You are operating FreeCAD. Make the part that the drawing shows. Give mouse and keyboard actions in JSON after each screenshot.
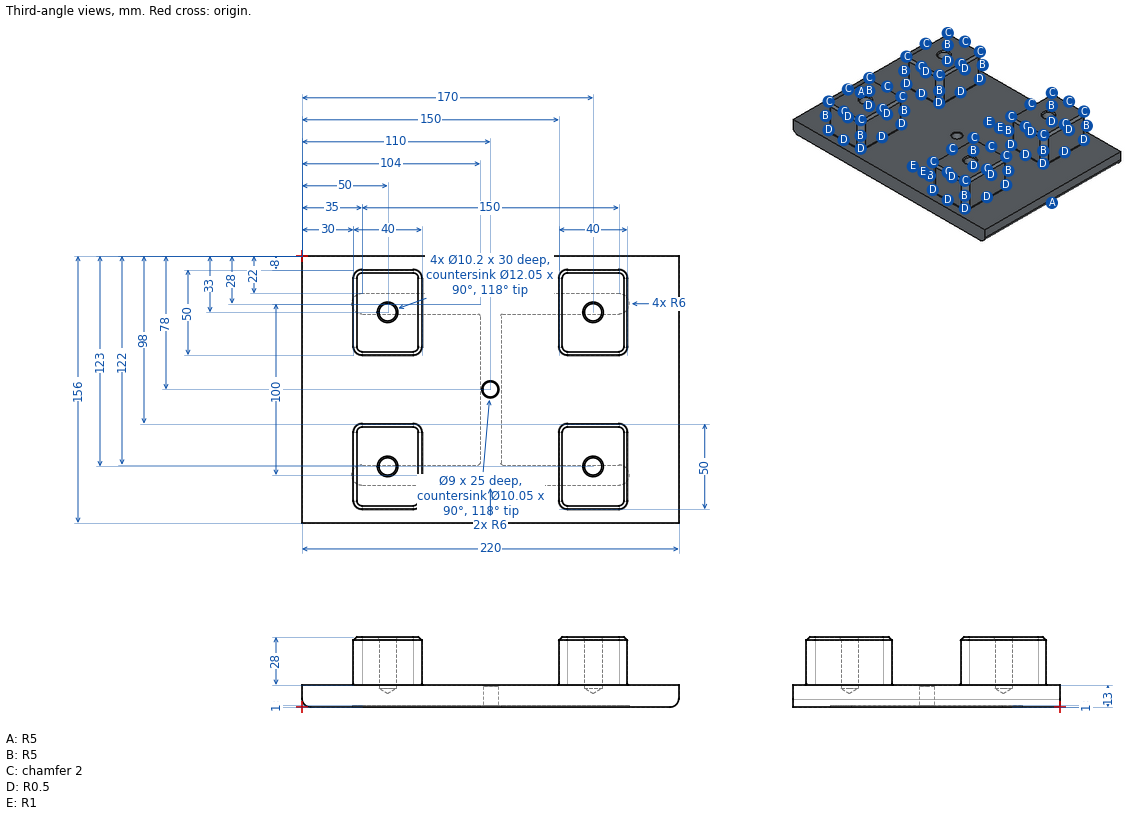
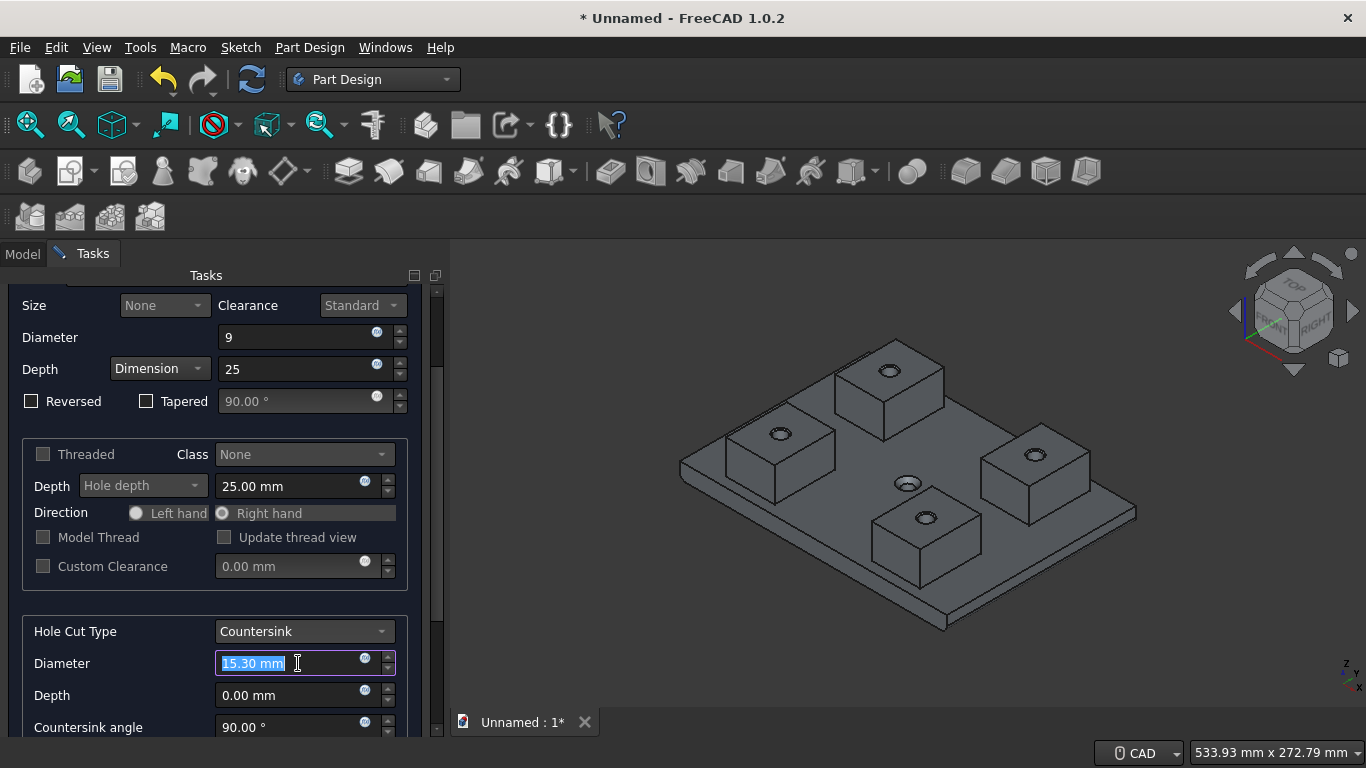
{"action": "type", "text": "10.05"}
{"action": "key", "text": "Tab"}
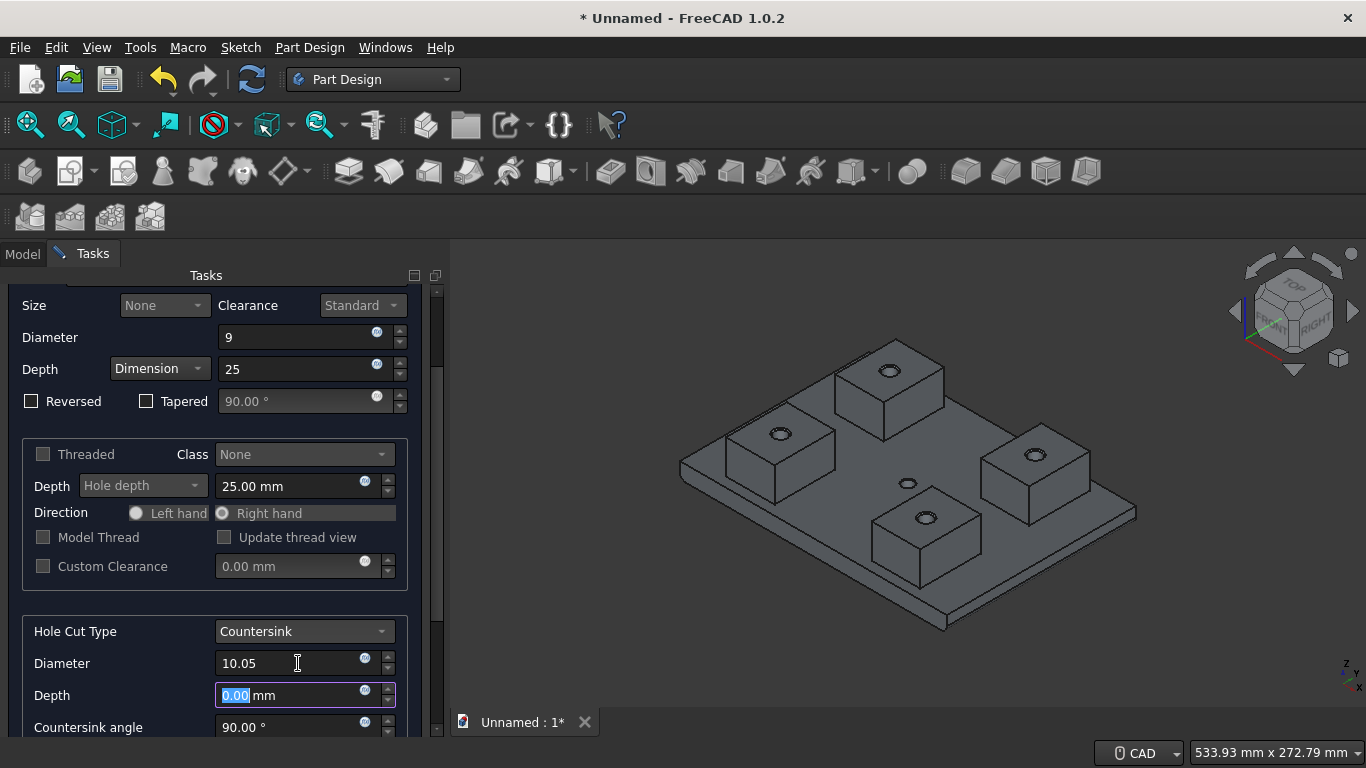
{"action": "scroll", "coordinate": [437, 510], "scroll_direction": "up", "scroll_amount": 3}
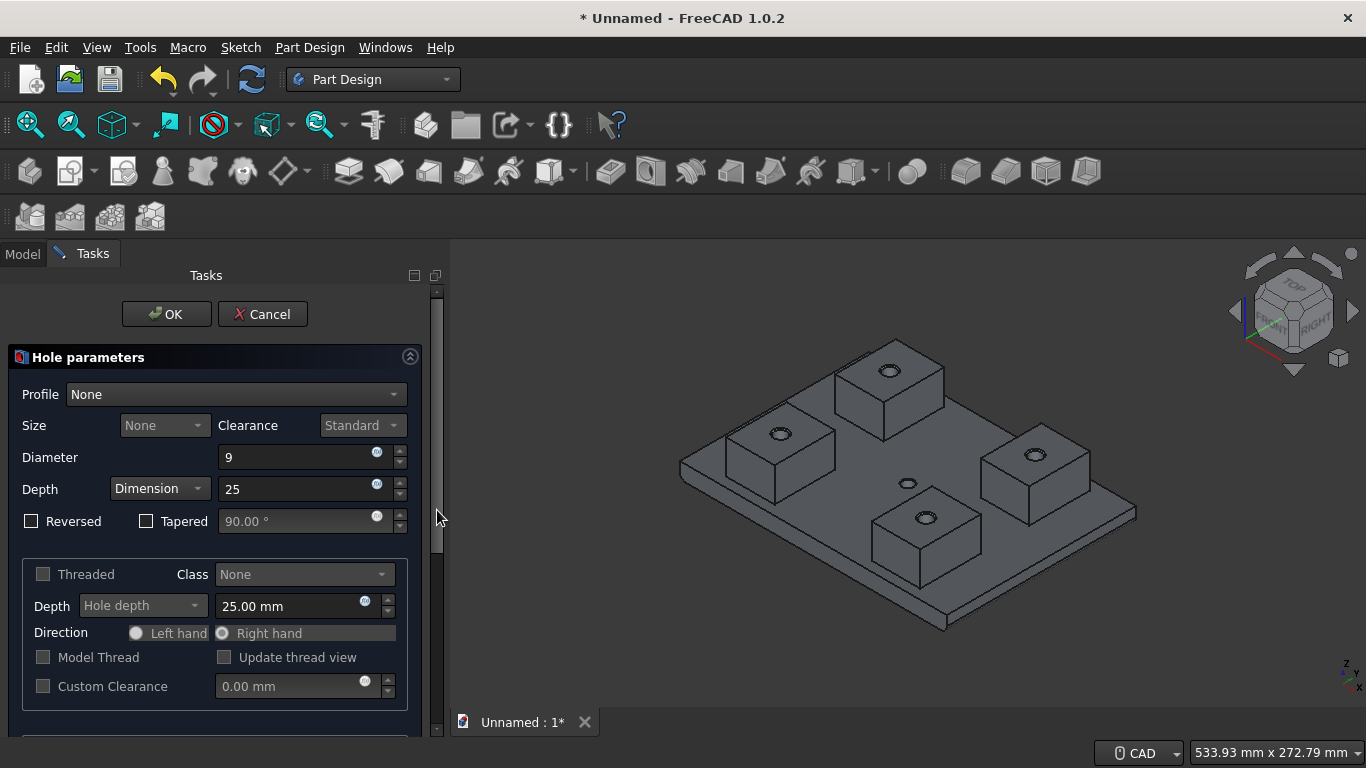
{"action": "left_click", "coordinate": [167, 314]}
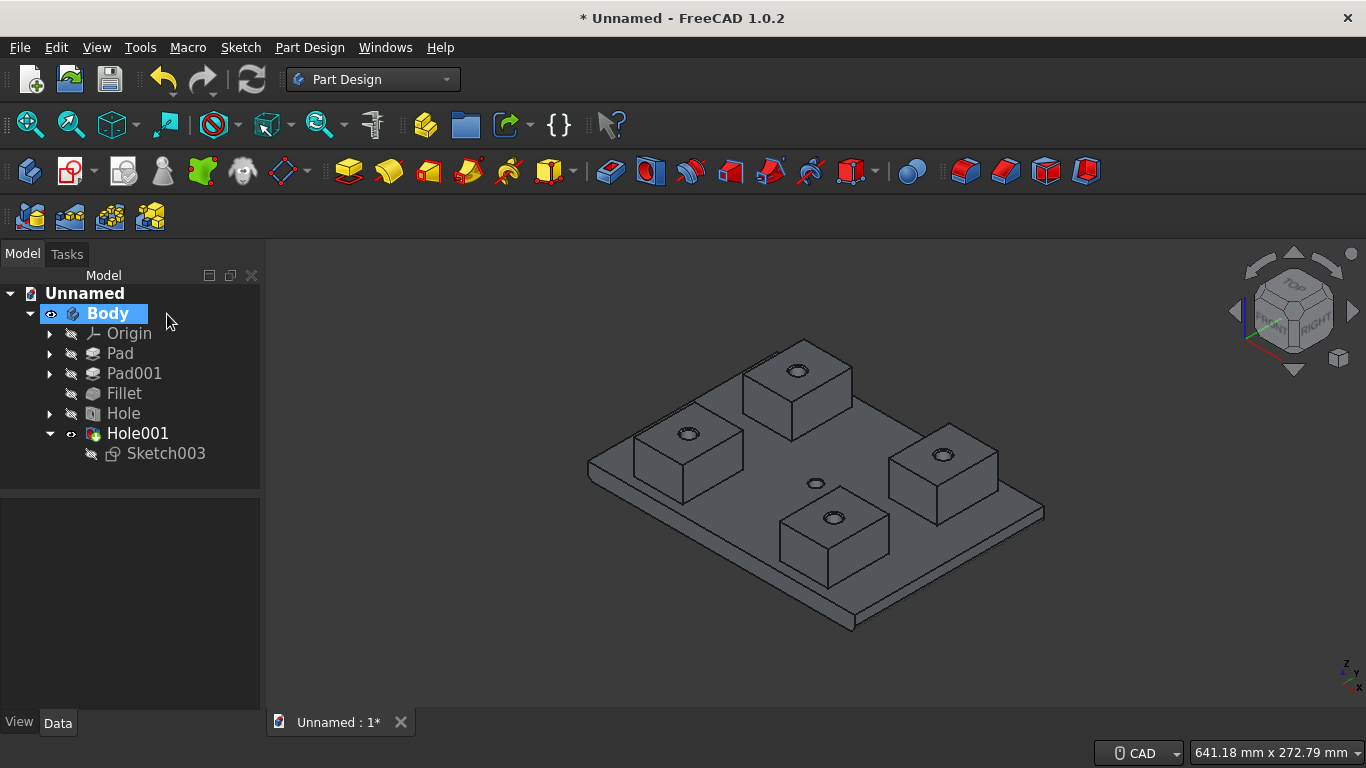
{"action": "left_click", "coordinate": [792, 421]}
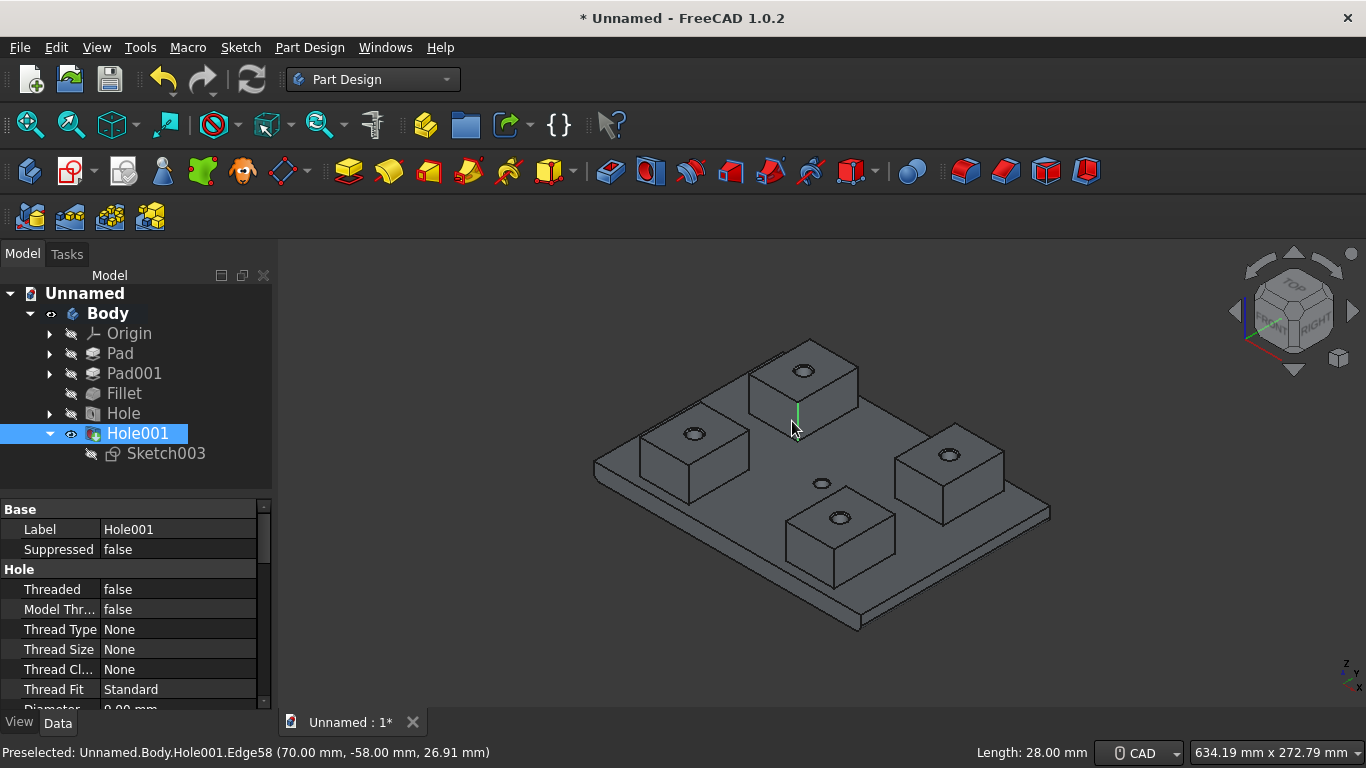
{"action": "left_click", "coordinate": [943, 505], "text": "ctrl"}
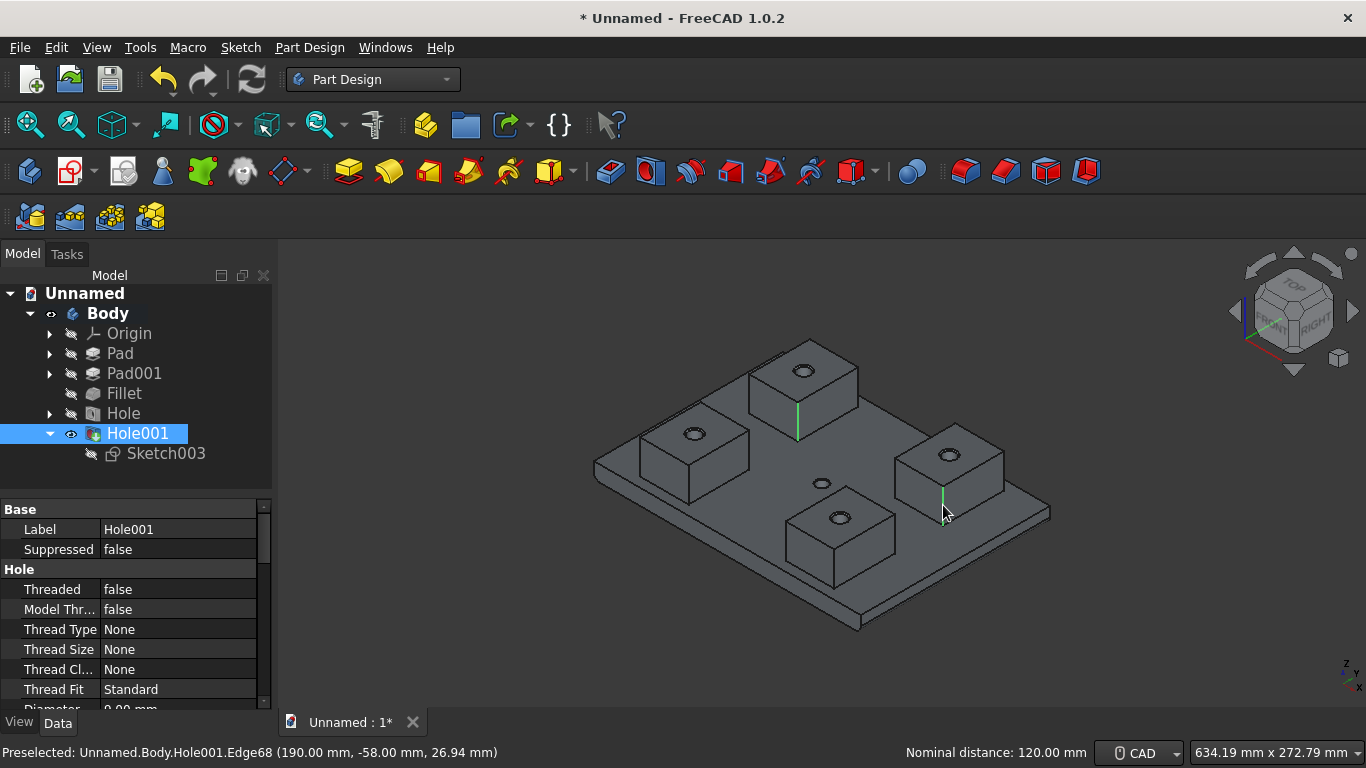
{"action": "left_click", "coordinate": [834, 568], "text": "ctrl"}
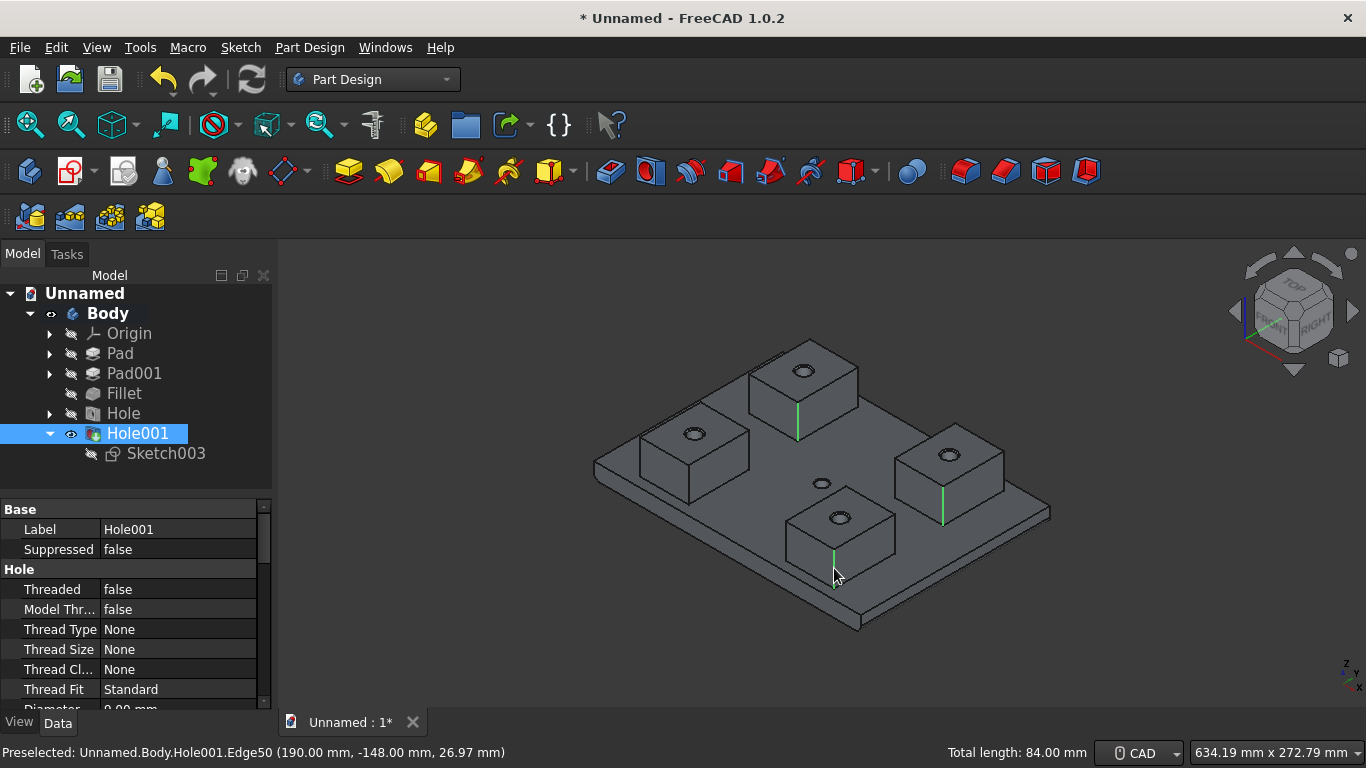
{"action": "left_click", "coordinate": [689, 484], "text": "ctrl"}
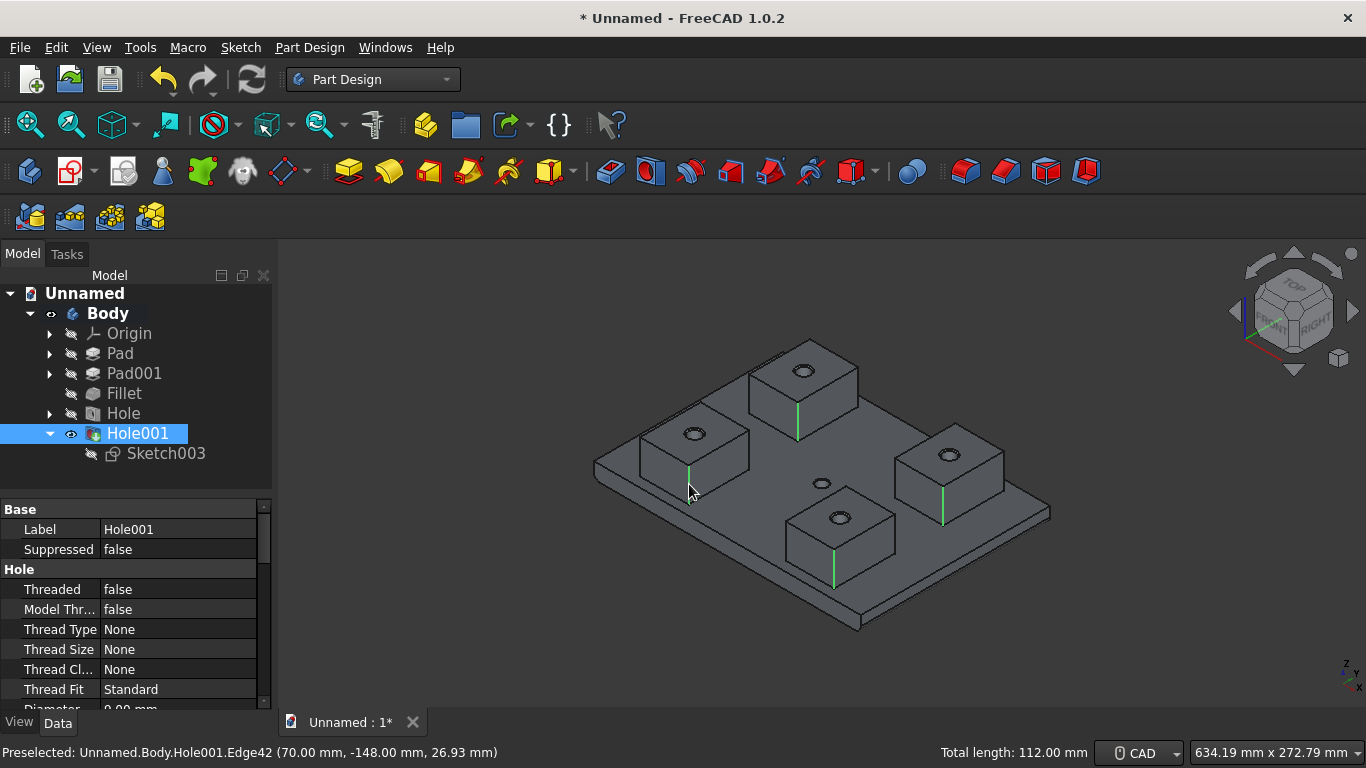
{"action": "key", "text": "2"}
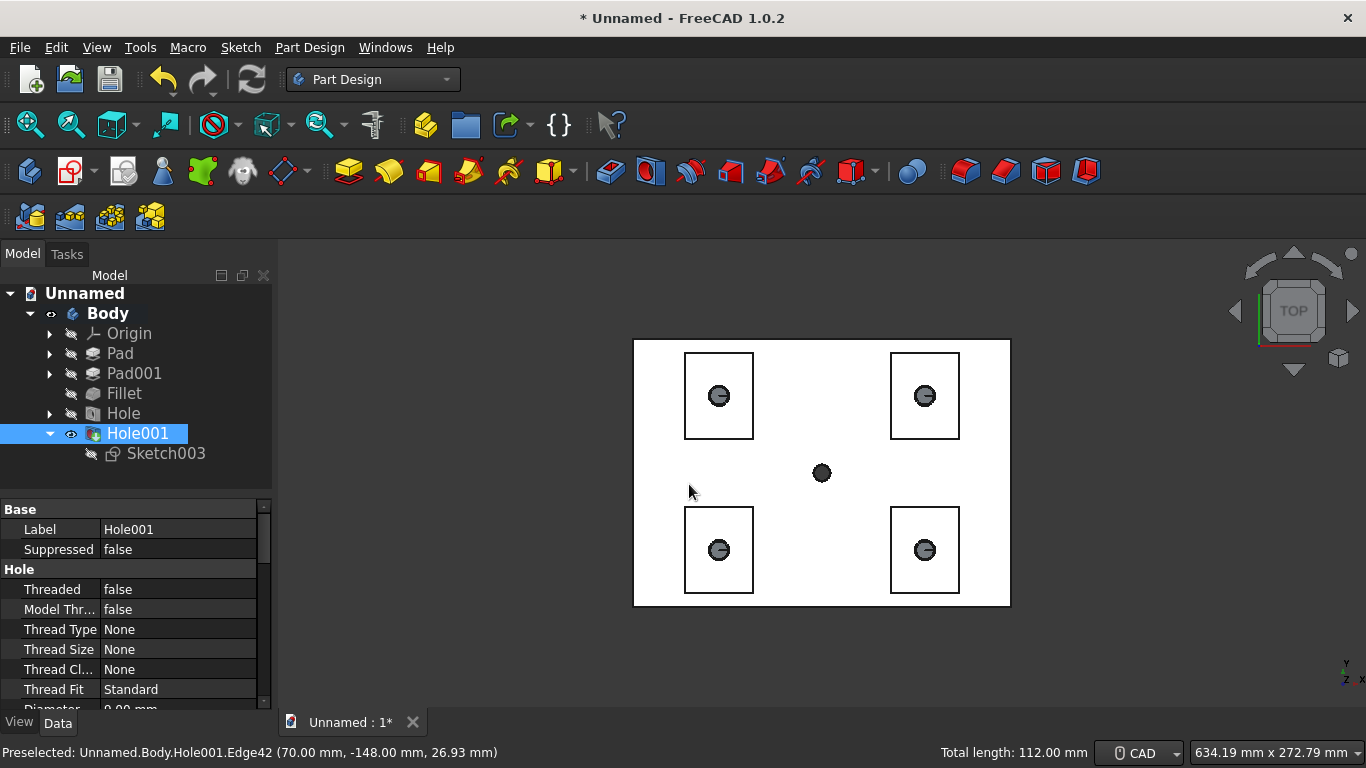
{"action": "key", "text": "0"}